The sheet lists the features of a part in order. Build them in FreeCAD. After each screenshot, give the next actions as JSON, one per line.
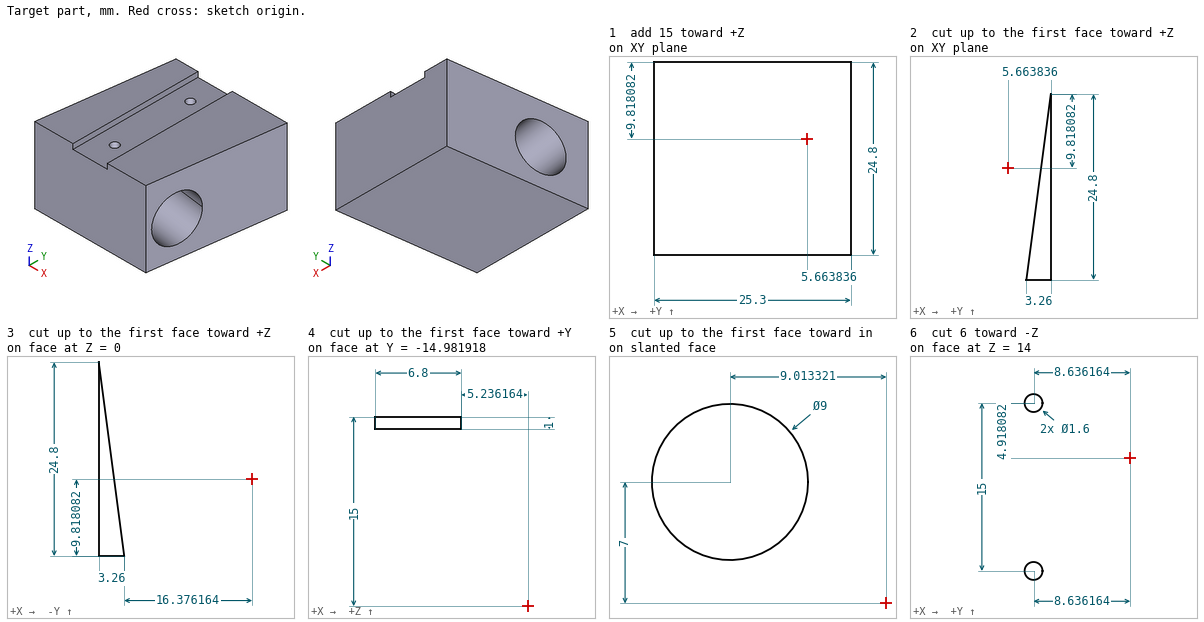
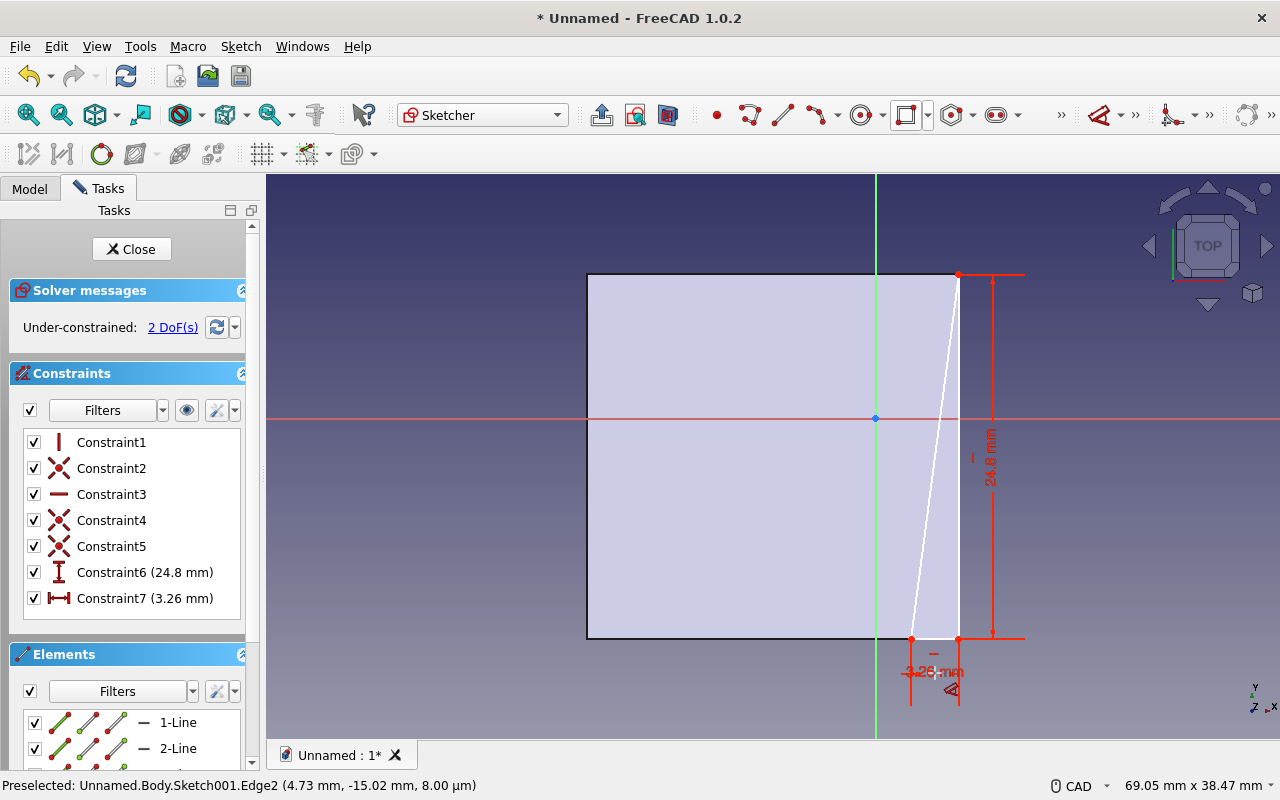
{"action": "left_click", "coordinate": [959, 275]}
{"action": "left_click", "coordinate": [917, 241]}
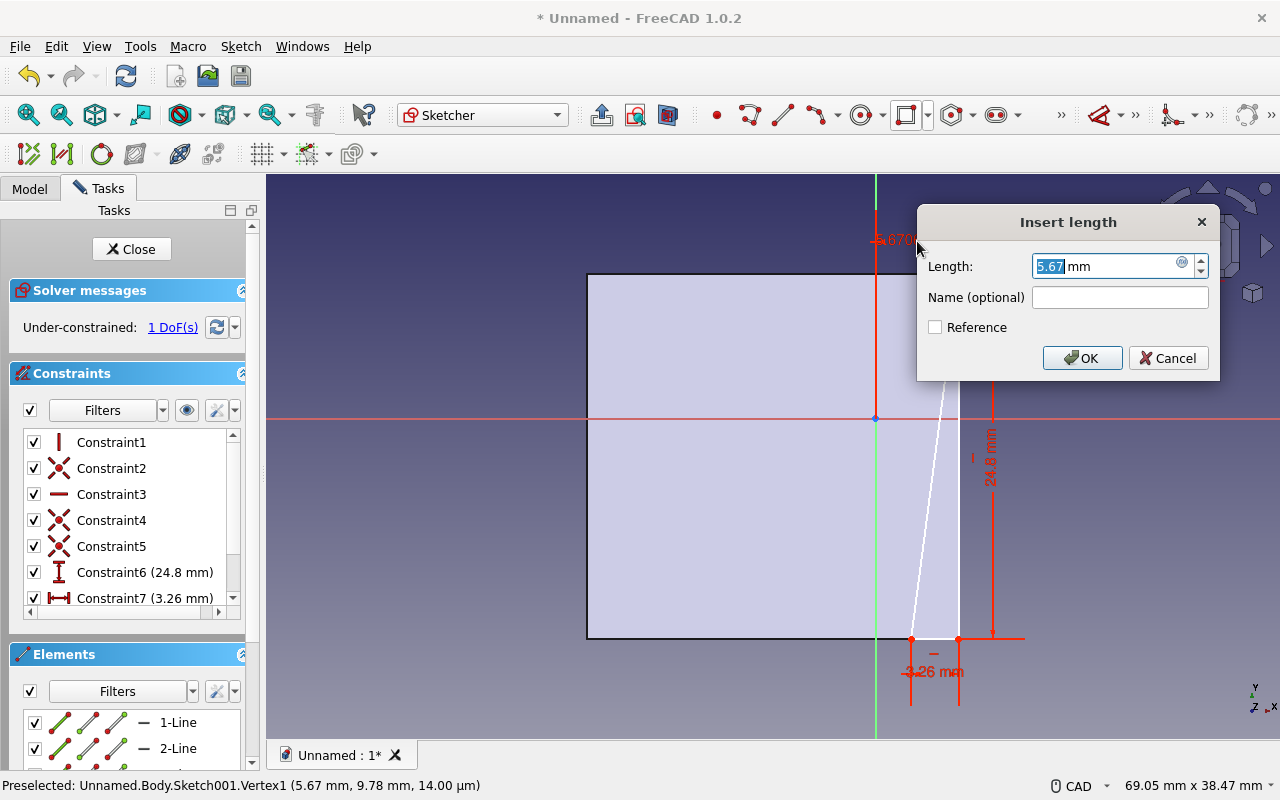
{"action": "type", "text": "5.663836"}
{"action": "key", "text": "Return"}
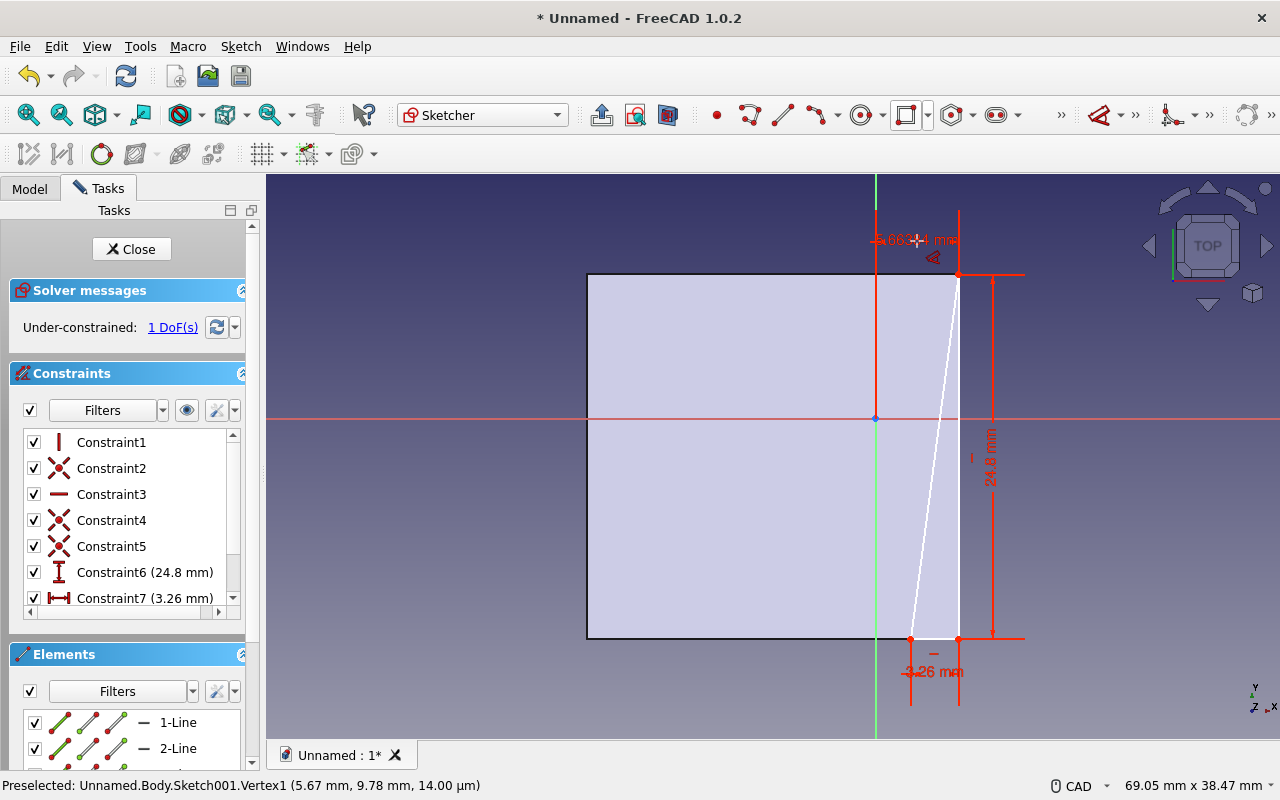
{"action": "left_click", "coordinate": [959, 275]}
{"action": "left_click", "coordinate": [993, 347]}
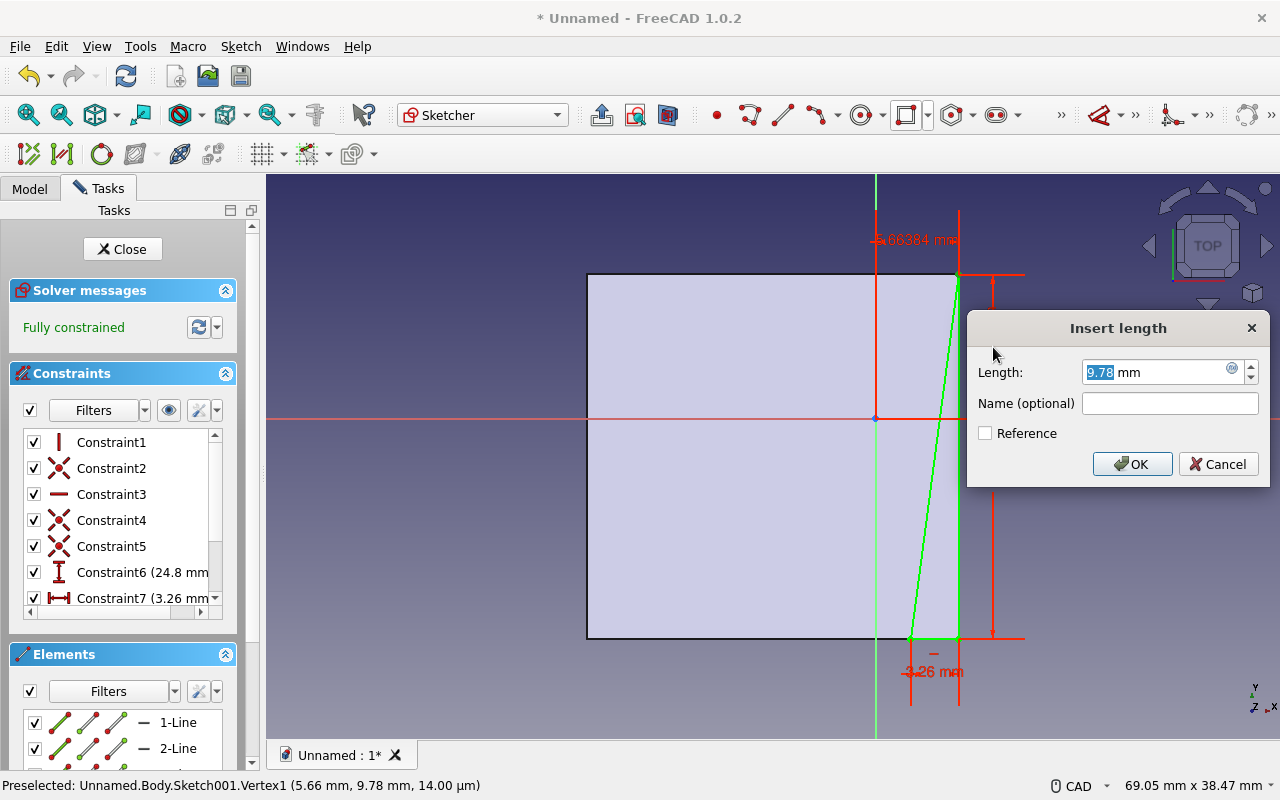
{"action": "type", "text": "9.818082"}
{"action": "key", "text": "Return"}
{"action": "key", "text": "Escape"}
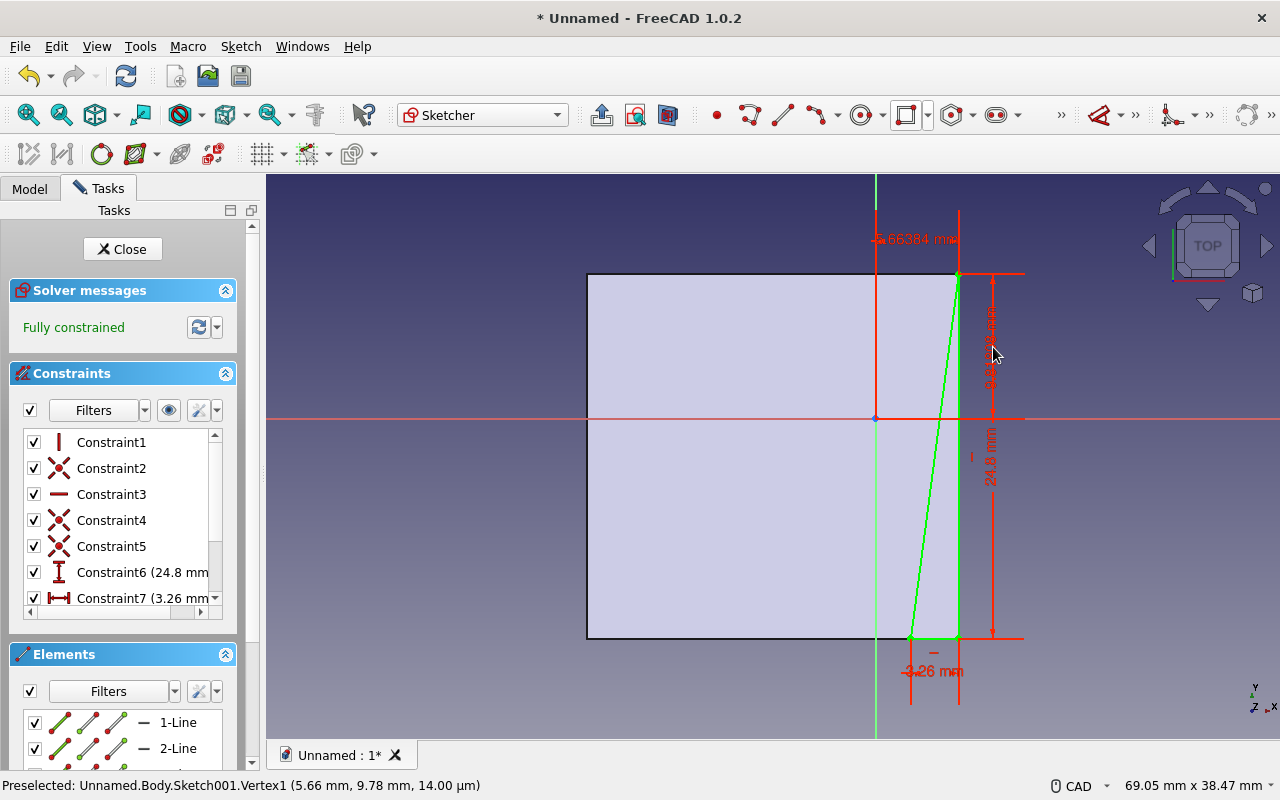
{"action": "left_click", "coordinate": [123, 249]}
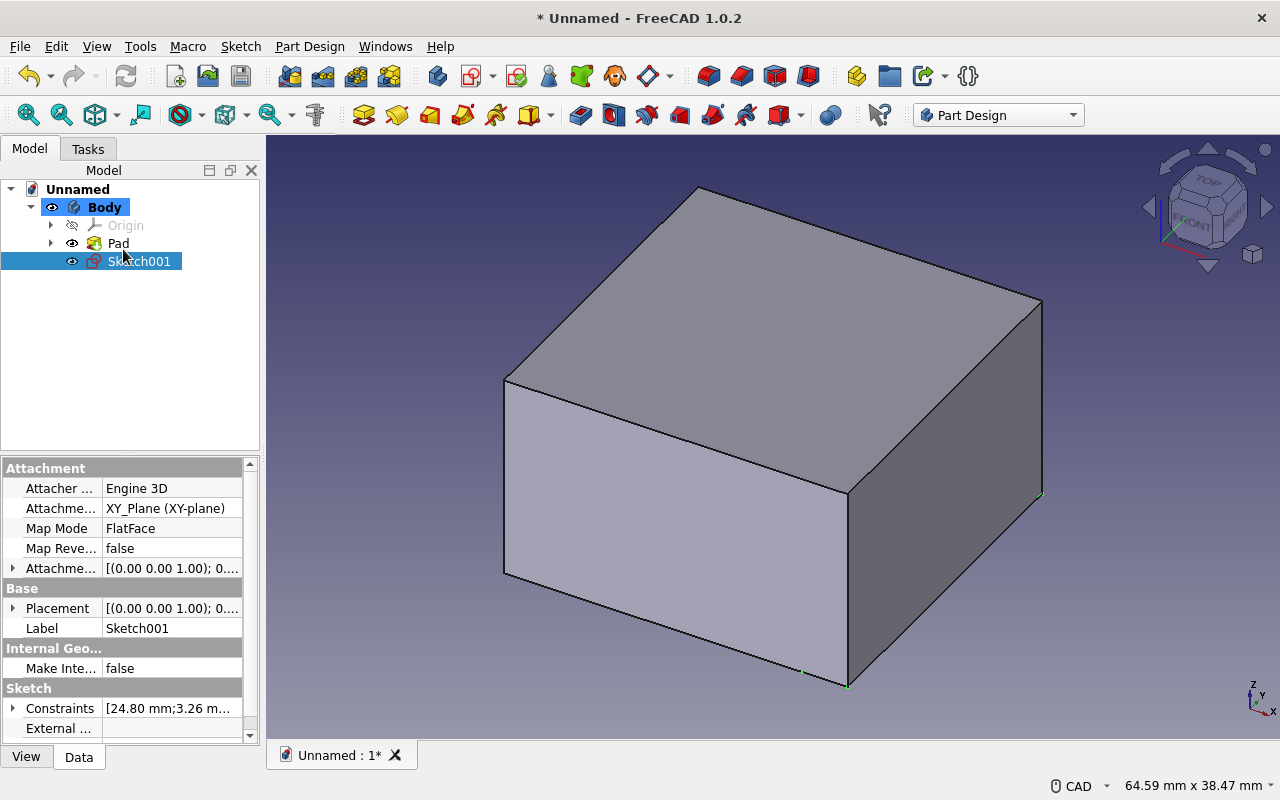
{"action": "left_click", "coordinate": [581, 116]}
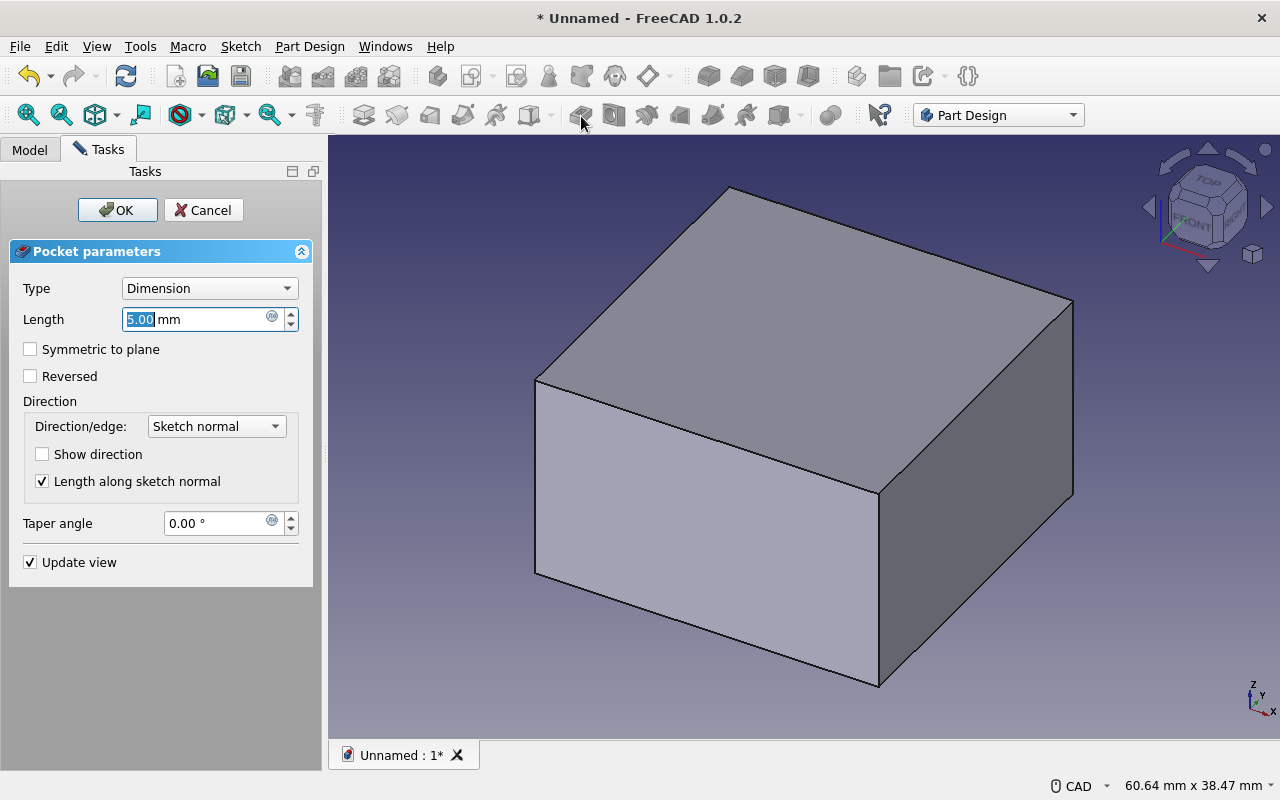
{"action": "left_click", "coordinate": [210, 288]}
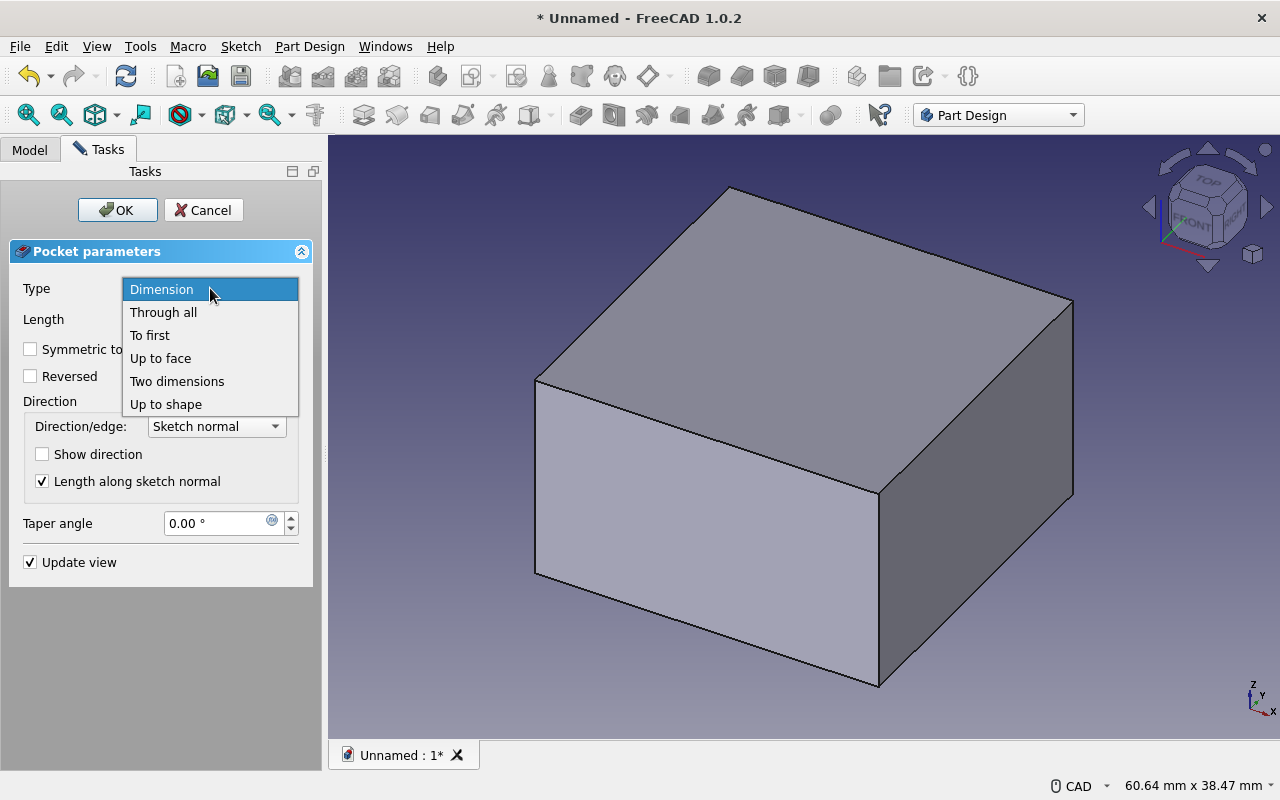
{"action": "left_click", "coordinate": [208, 336]}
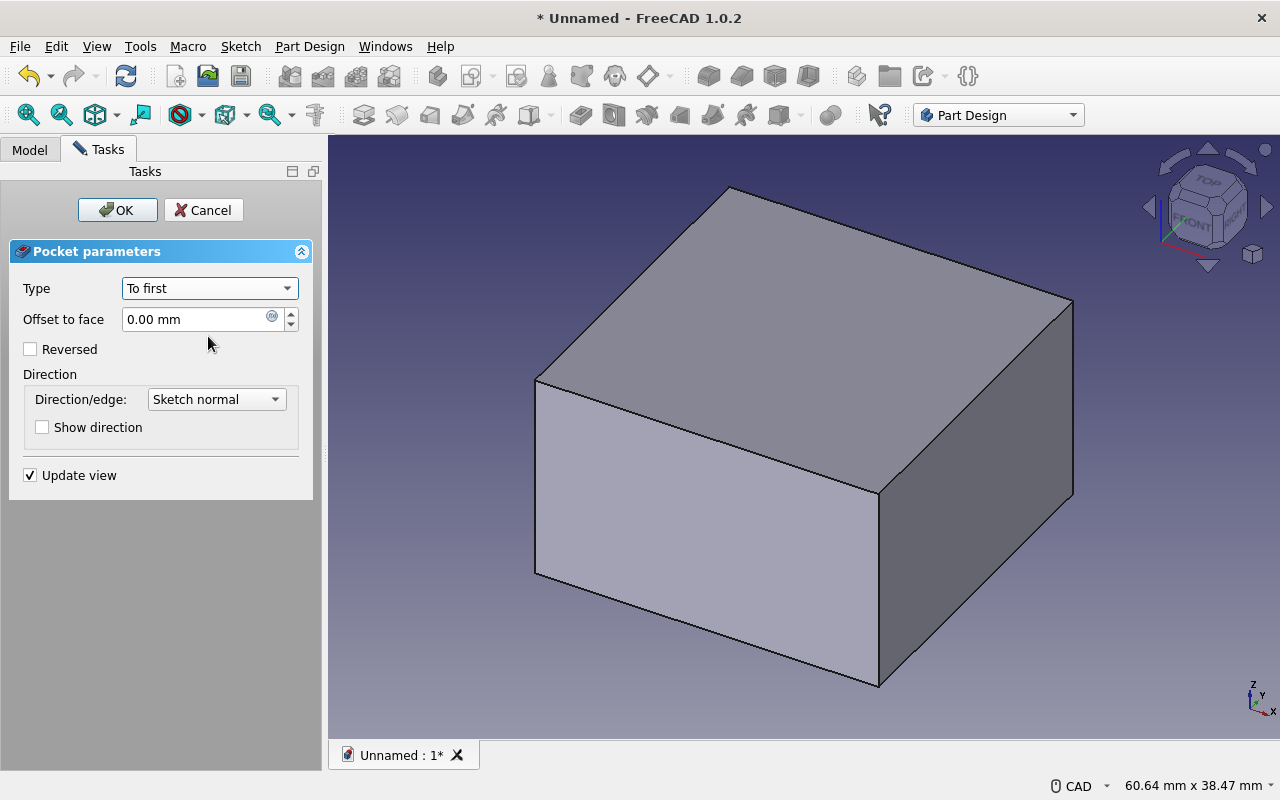
{"action": "left_click", "coordinate": [31, 349]}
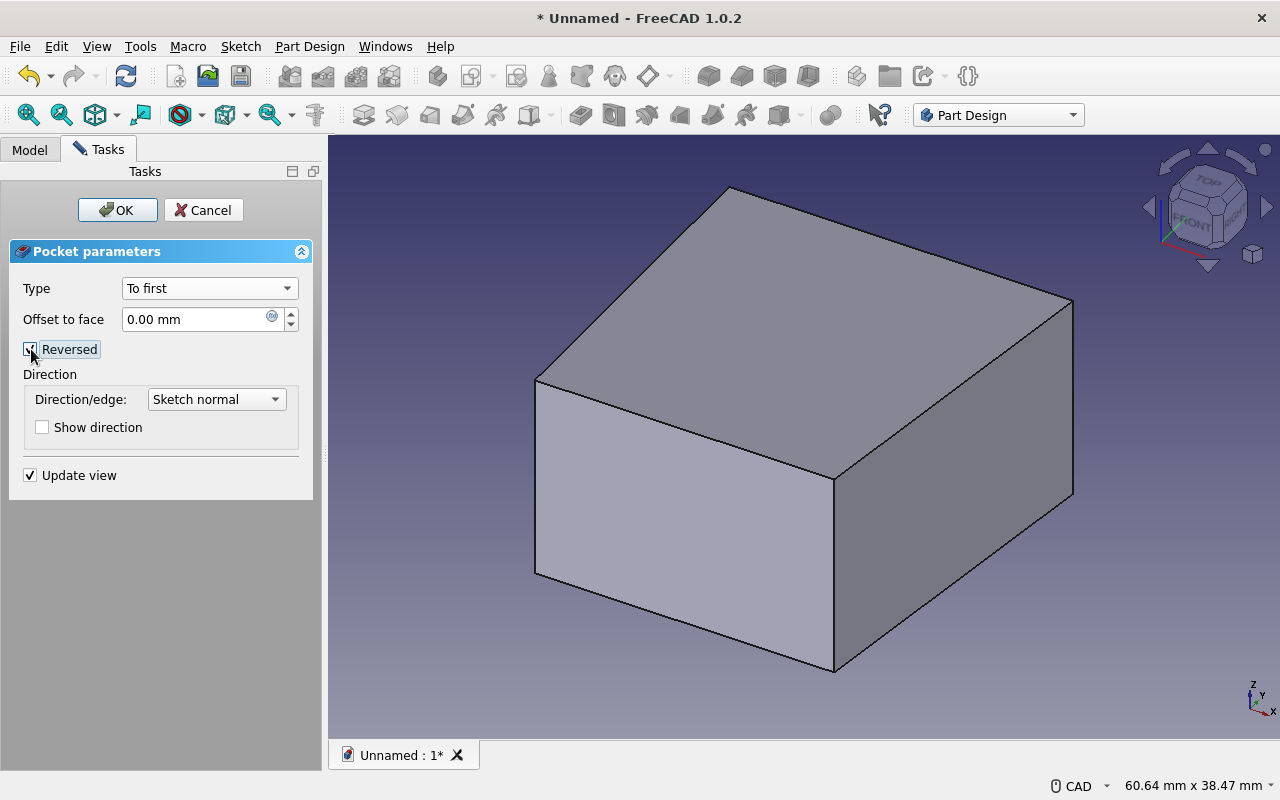
{"action": "left_click", "coordinate": [118, 210]}